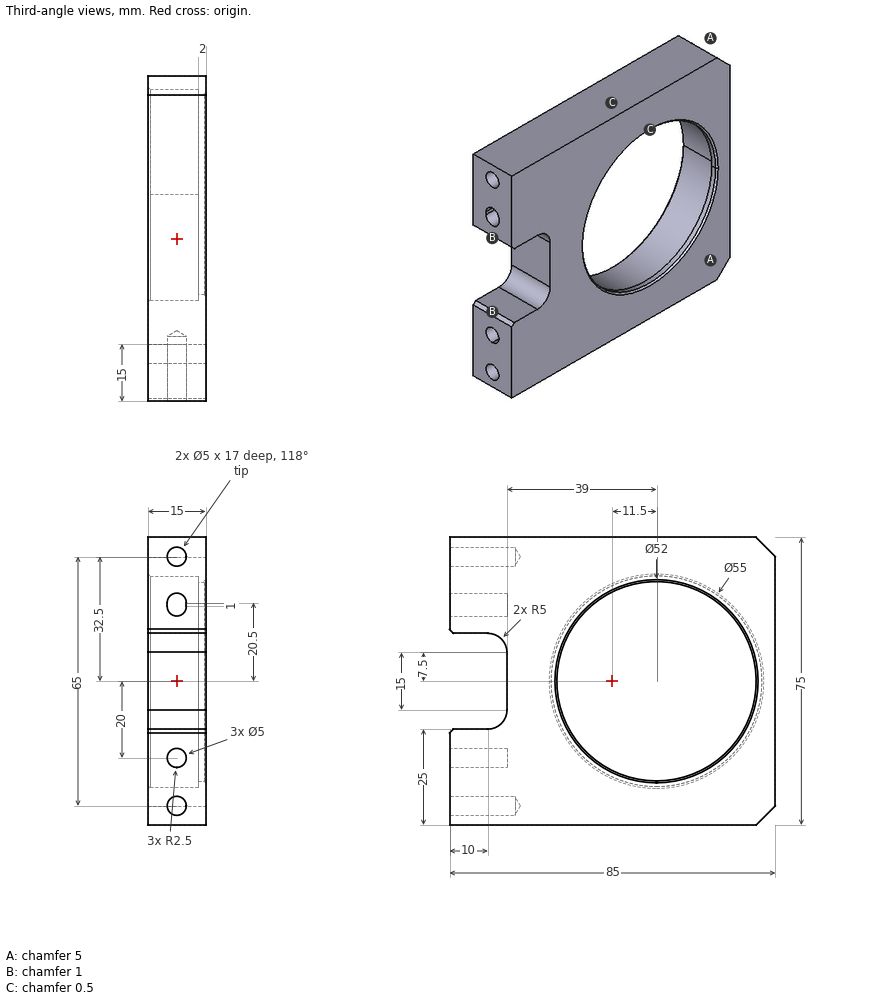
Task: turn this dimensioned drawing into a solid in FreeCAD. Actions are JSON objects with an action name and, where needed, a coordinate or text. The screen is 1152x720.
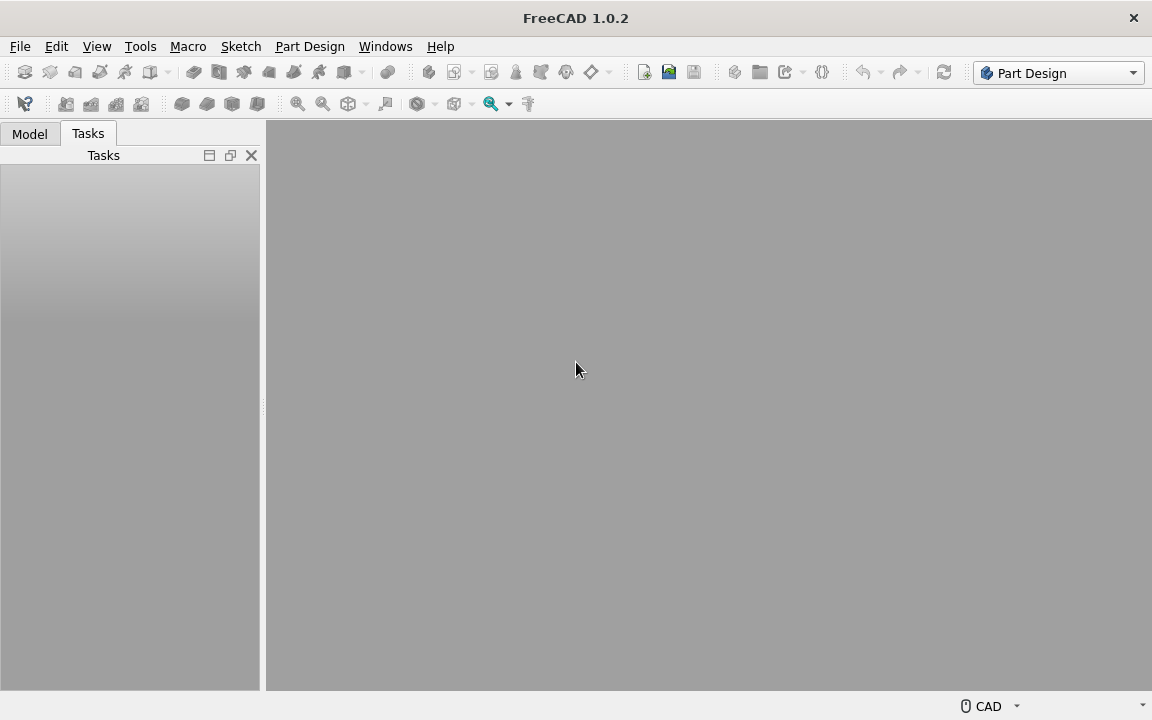
{"action": "left_click", "coordinate": [644, 72]}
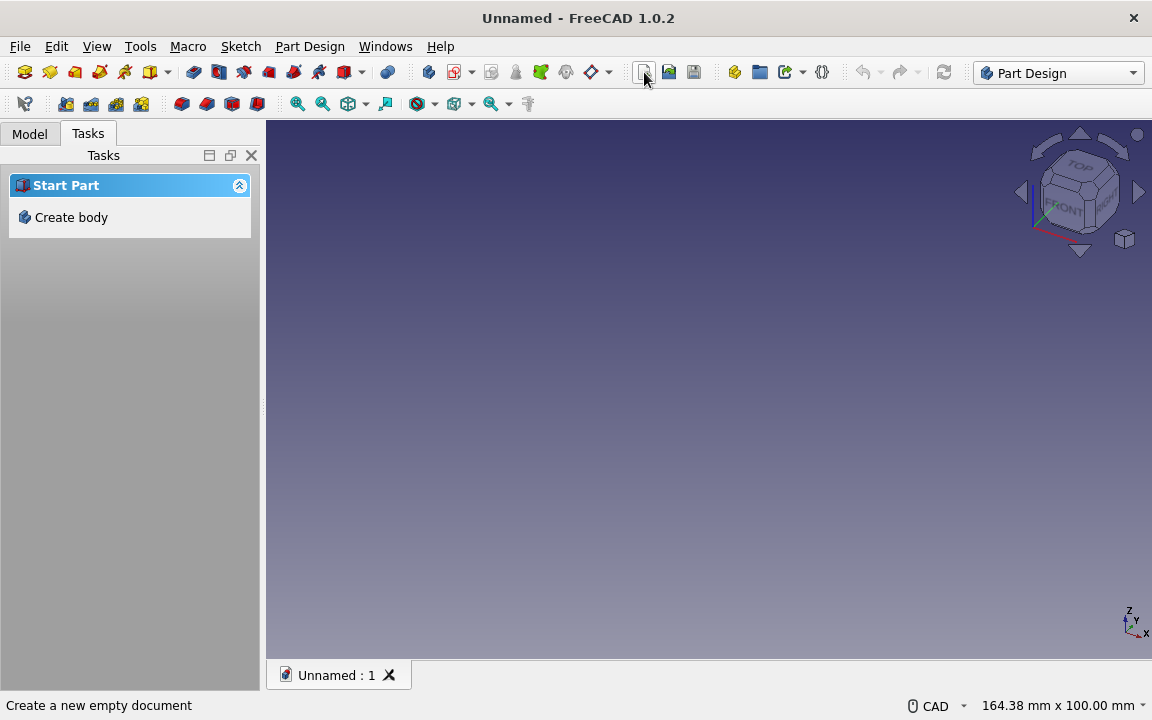
{"action": "left_click", "coordinate": [454, 72]}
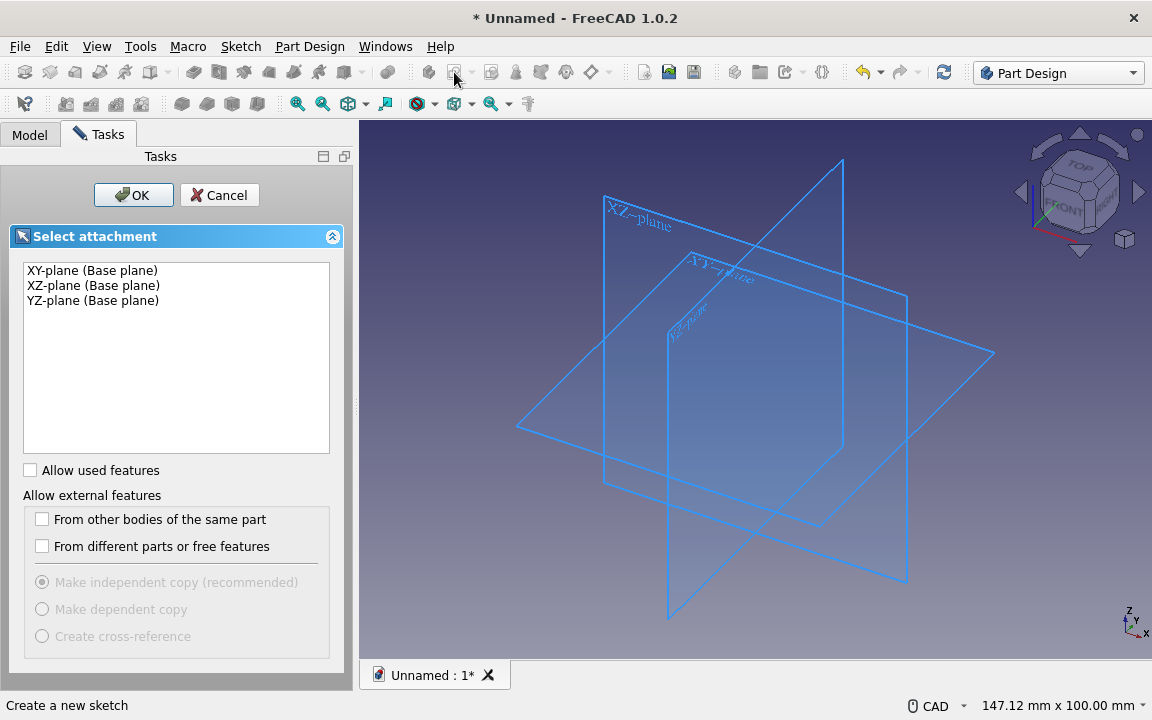
{"action": "left_click", "coordinate": [84, 300]}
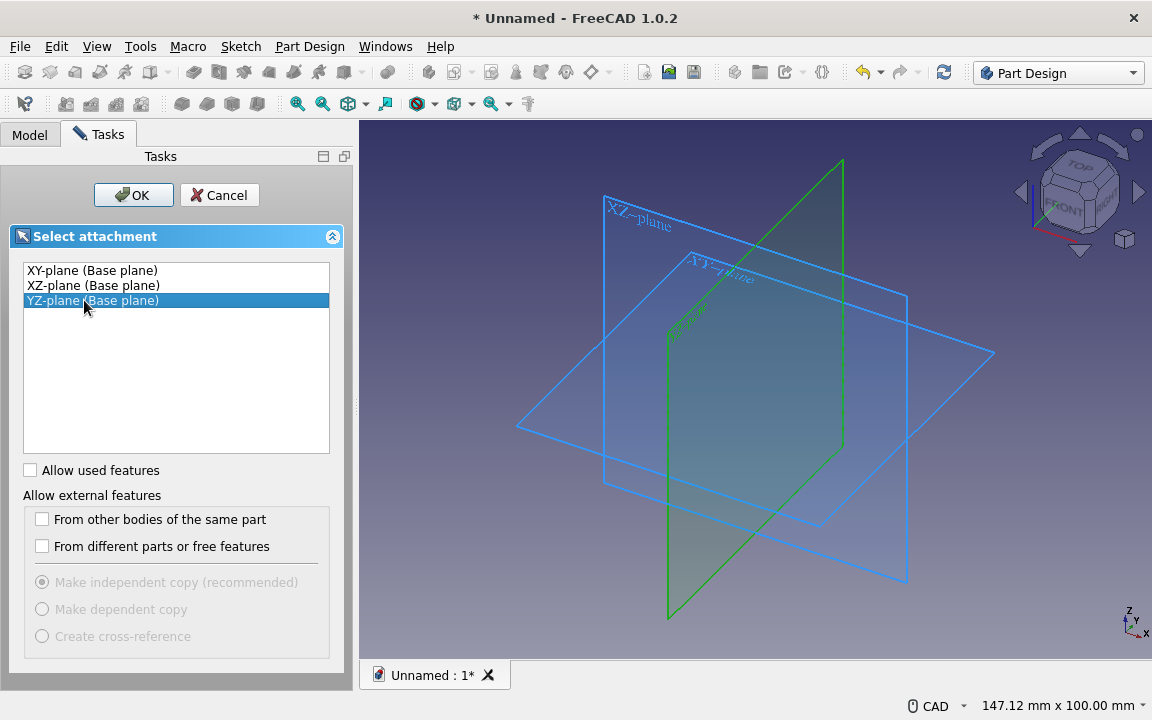
{"action": "left_click", "coordinate": [134, 195]}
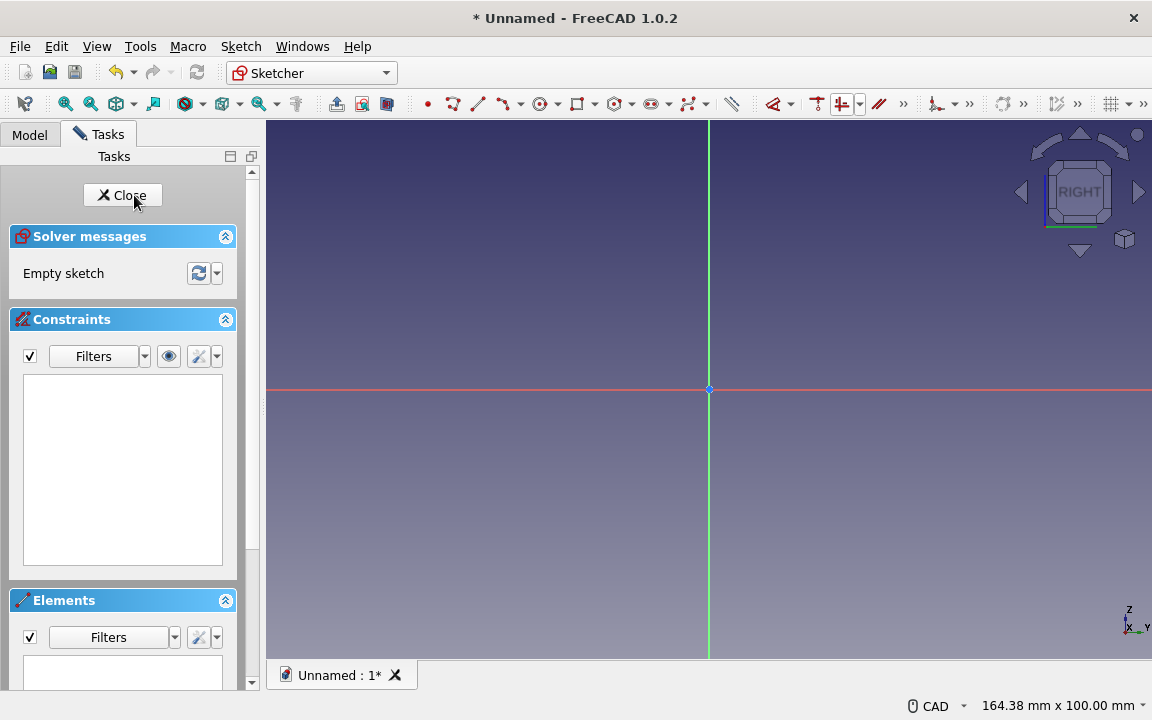
{"action": "left_click", "coordinate": [478, 104]}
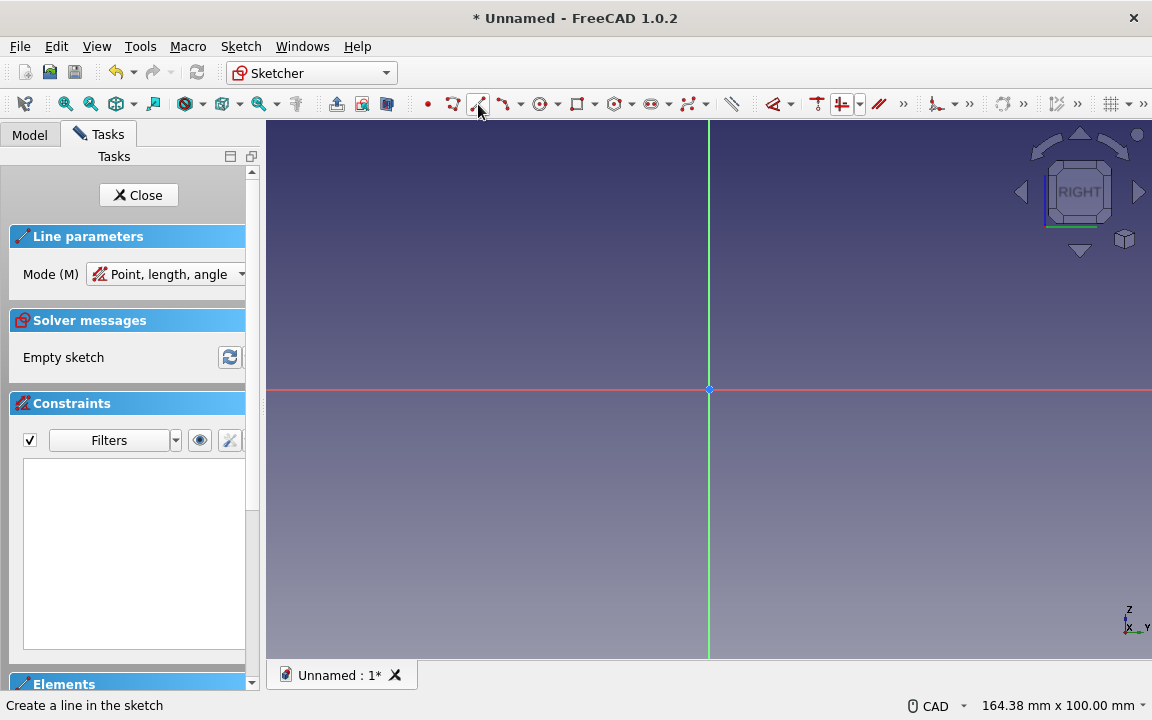
{"action": "left_click", "coordinate": [561, 349]}
{"action": "left_click", "coordinate": [561, 430]}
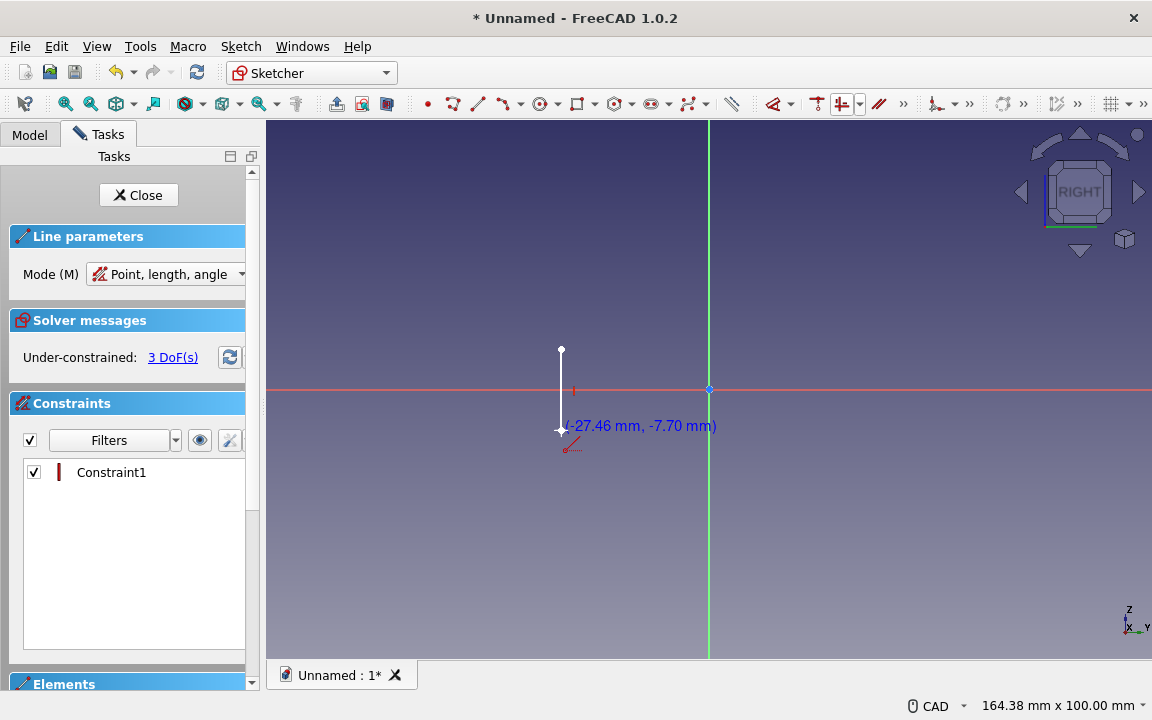
{"action": "left_click", "coordinate": [453, 104]}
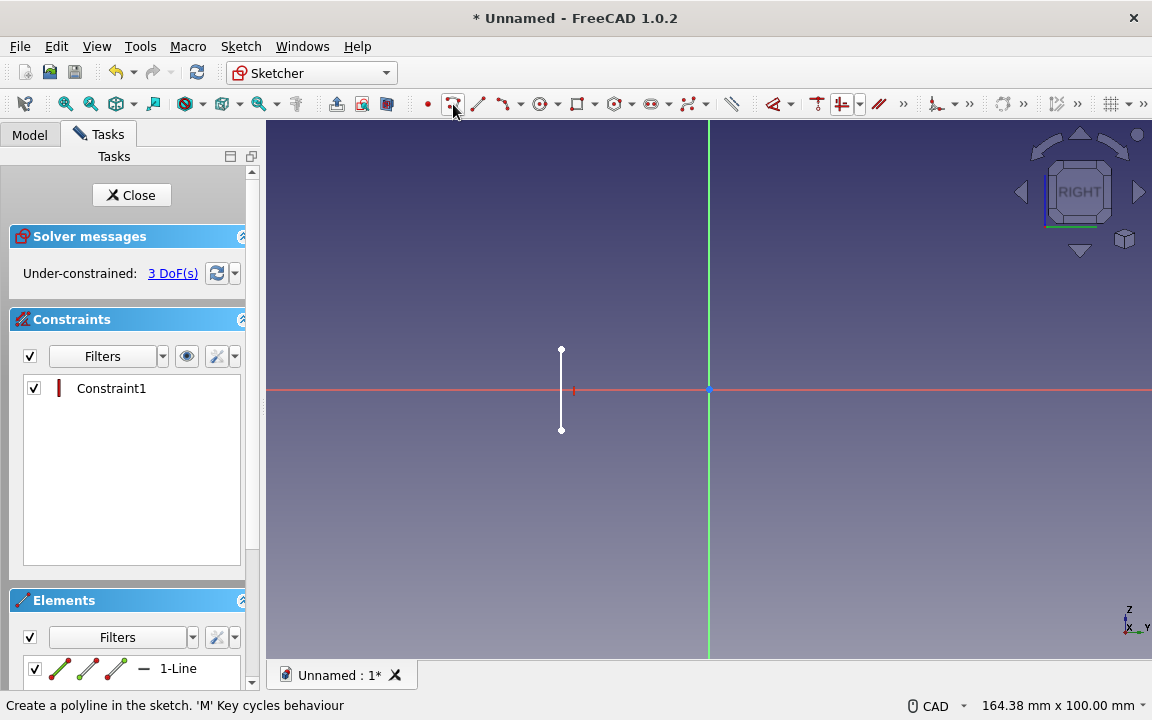
{"action": "left_click", "coordinate": [534, 457]}
{"action": "left_click", "coordinate": [480, 457]}
{"action": "left_click", "coordinate": [480, 592]}
{"action": "left_click", "coordinate": [938, 592]}
{"action": "left_click", "coordinate": [938, 187]}
{"action": "left_click", "coordinate": [480, 187]}
{"action": "left_click", "coordinate": [480, 322]}
{"action": "left_click", "coordinate": [534, 322]}
{"action": "right_click", "coordinate": [534, 322]}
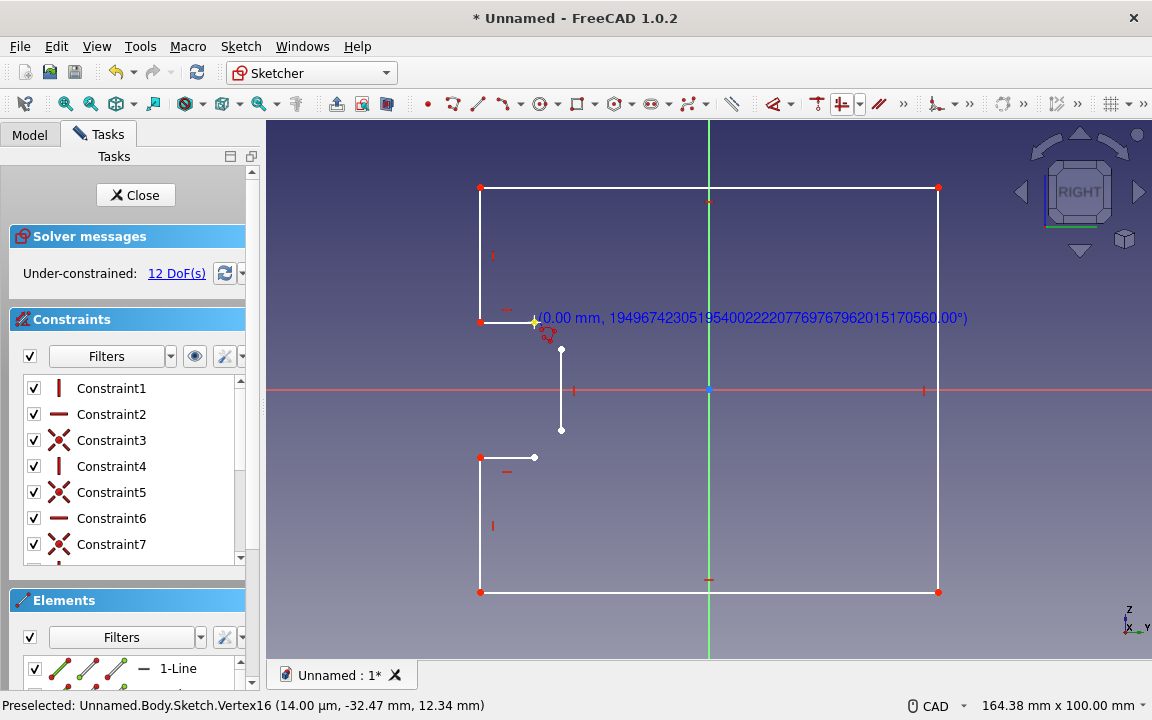
{"action": "left_click", "coordinate": [502, 104]}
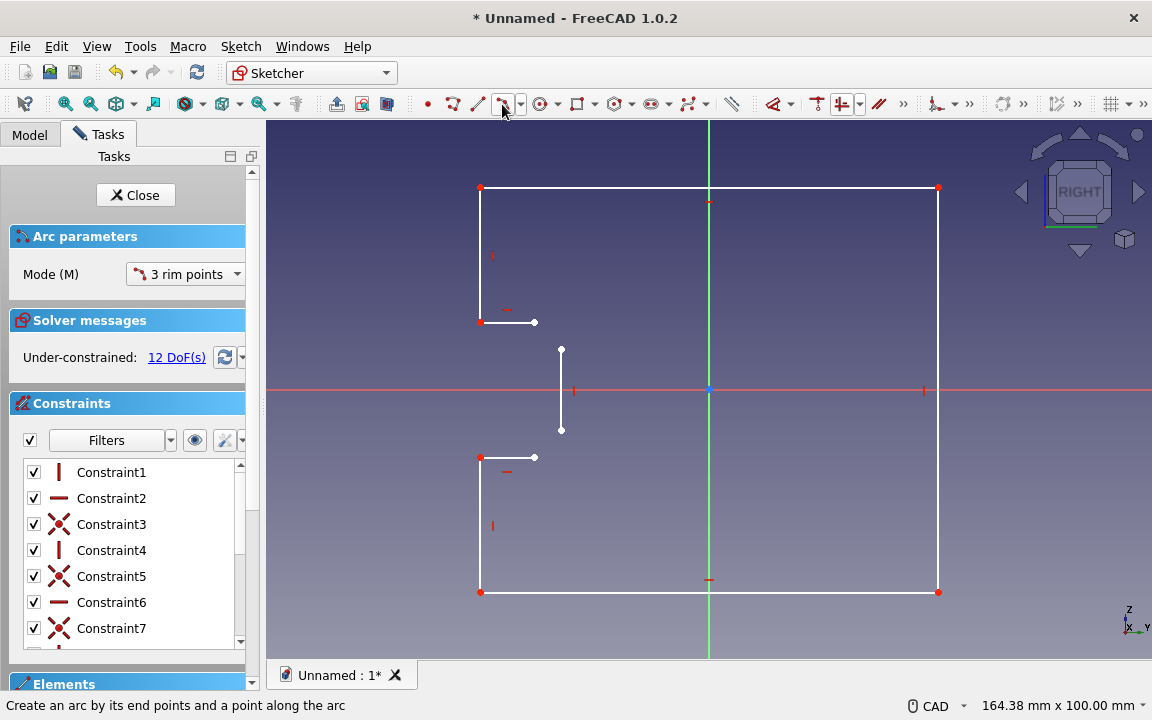
{"action": "left_click", "coordinate": [561, 431]}
{"action": "left_click", "coordinate": [534, 458]}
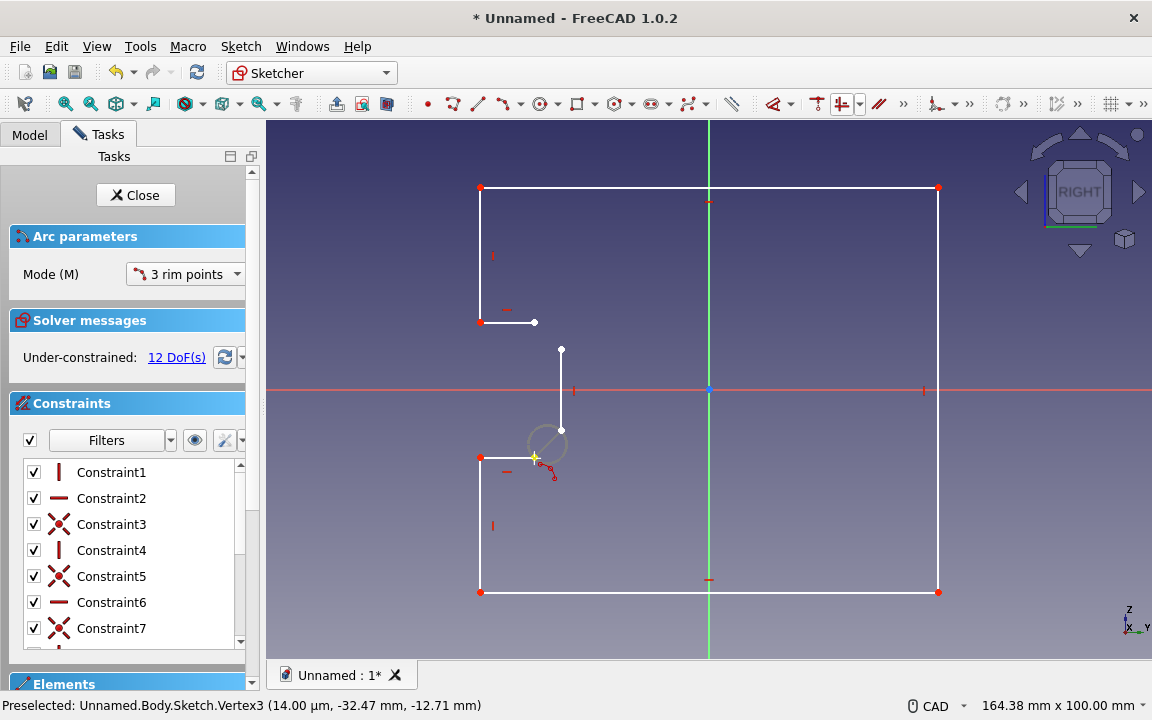
{"action": "scroll", "coordinate": [553, 449], "scroll_direction": "up", "scroll_amount": 4}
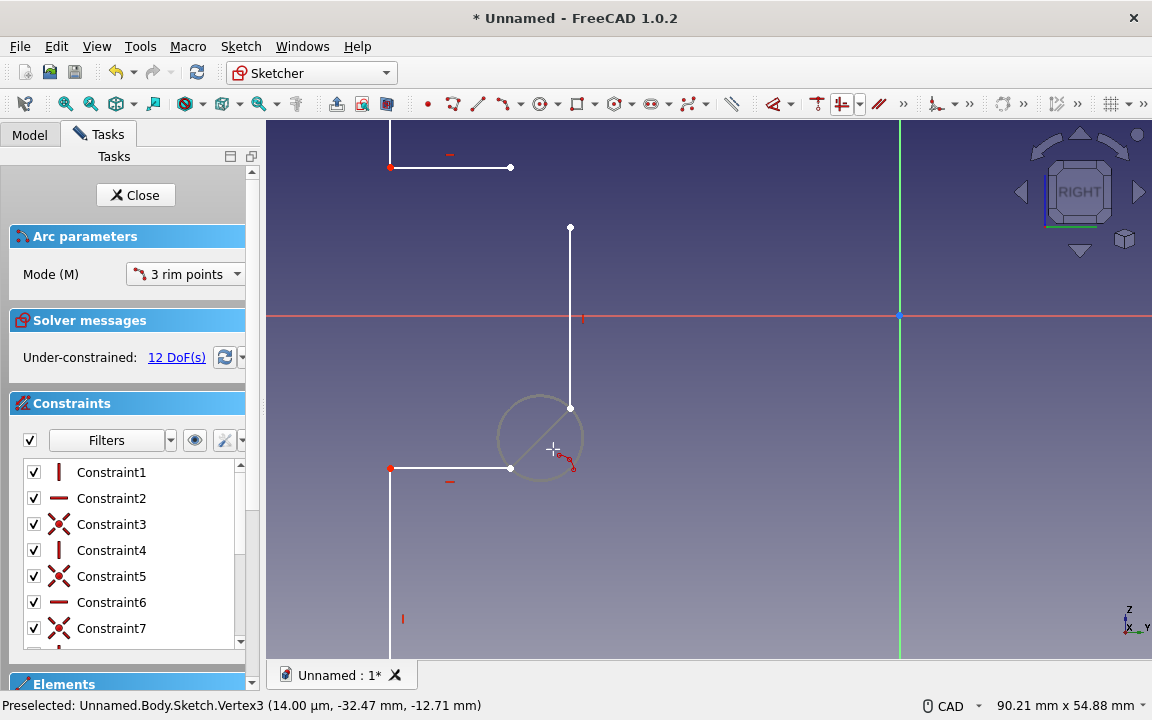
{"action": "left_click", "coordinate": [552, 448]}